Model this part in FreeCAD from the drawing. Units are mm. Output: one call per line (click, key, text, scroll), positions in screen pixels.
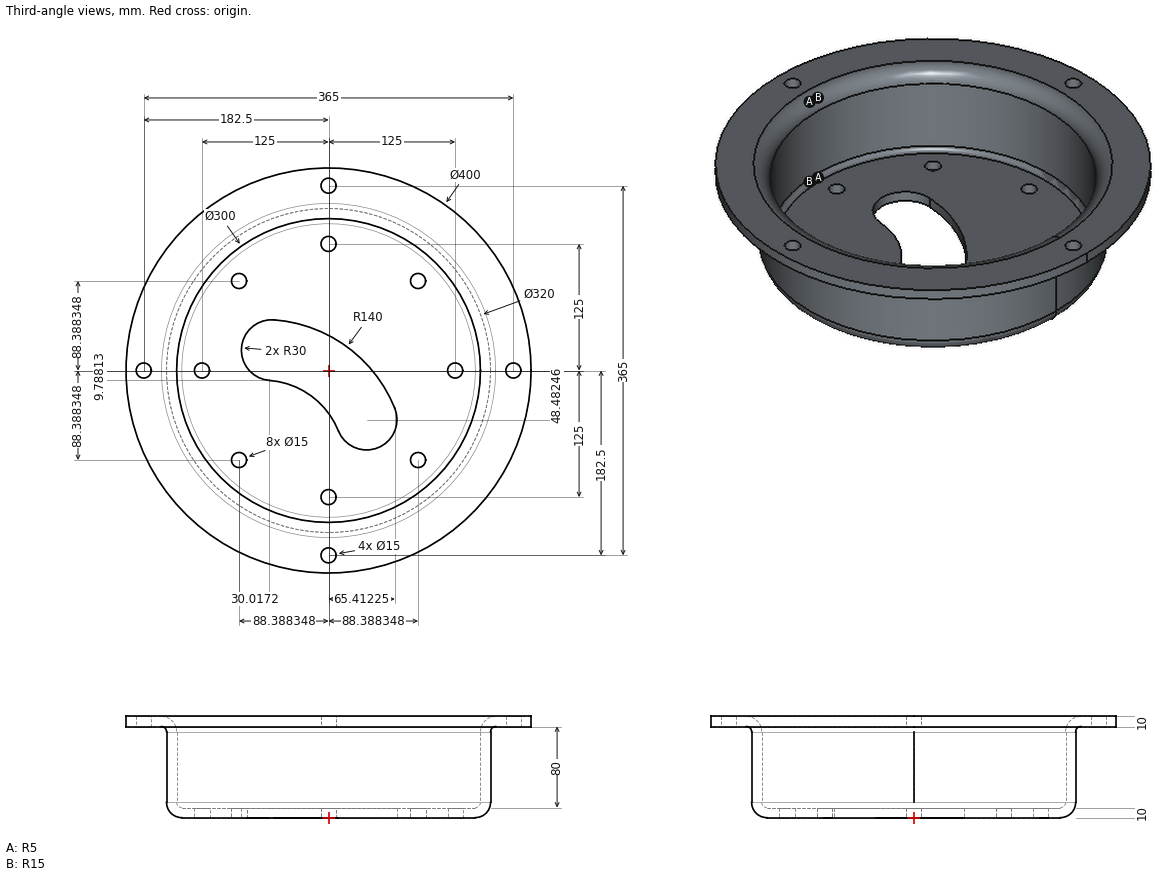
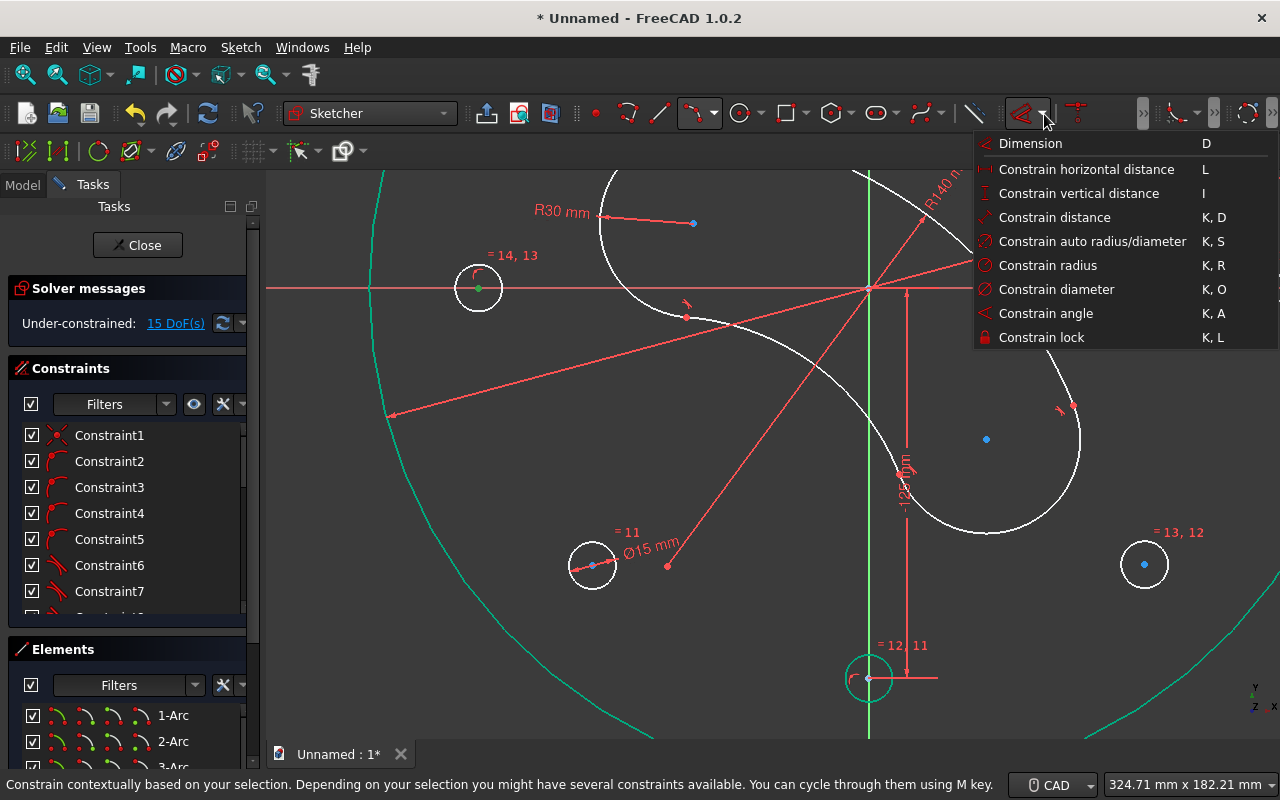
click(1126, 169)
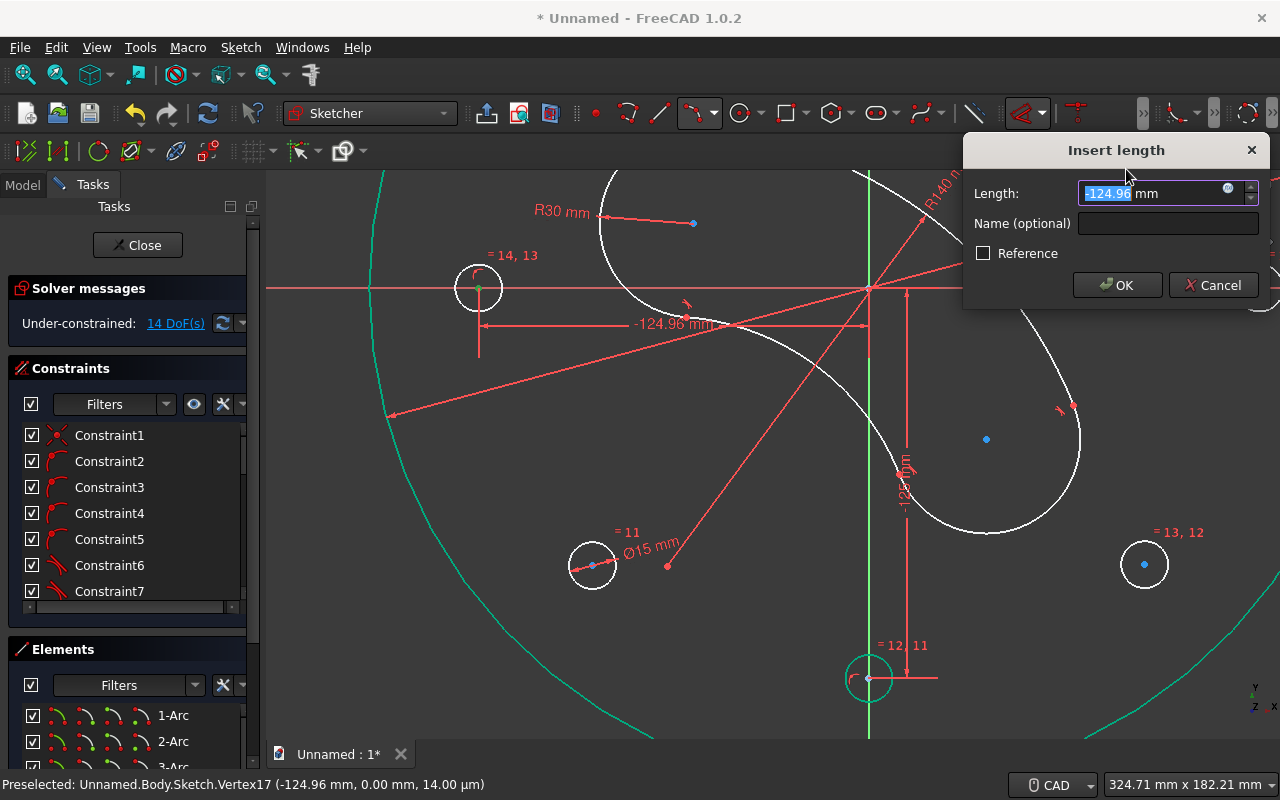
text(-125)
key(Return)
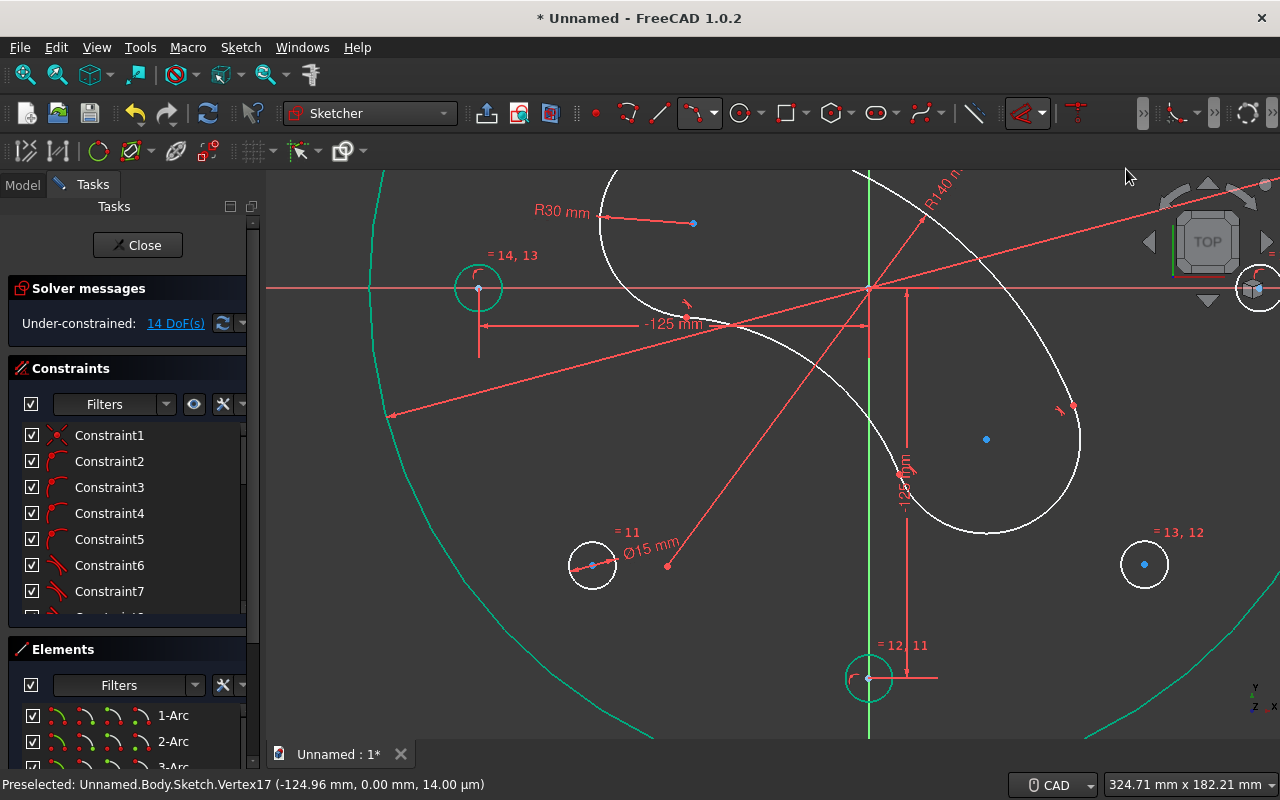
scroll(609, 551, down, 5)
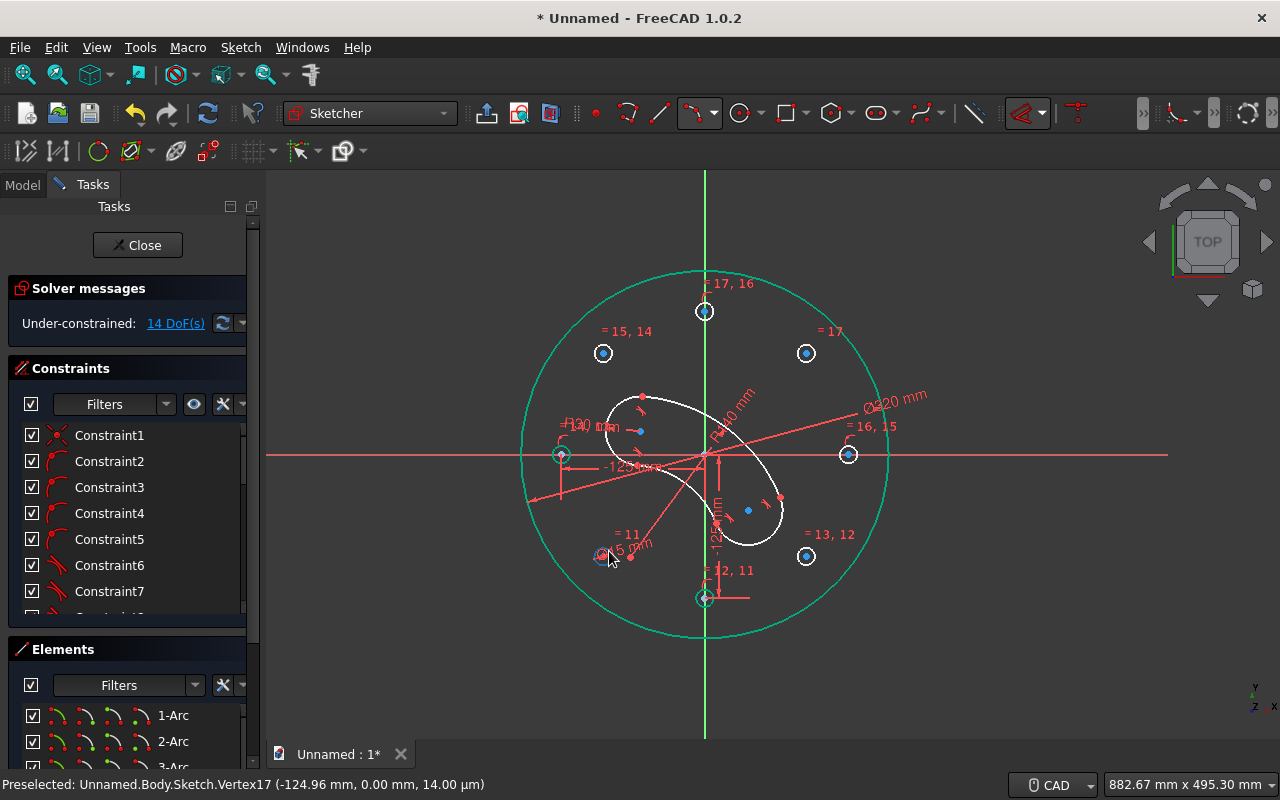
click(849, 455)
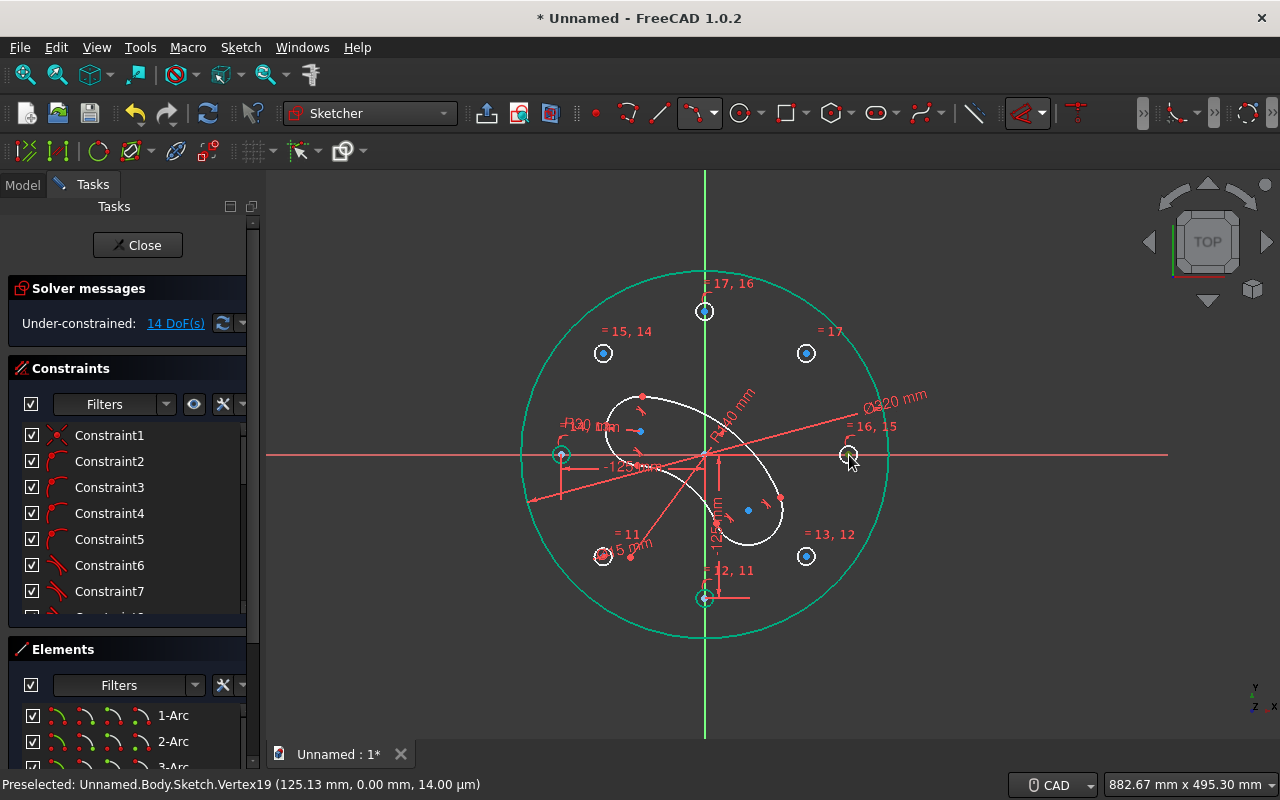
click(1044, 114)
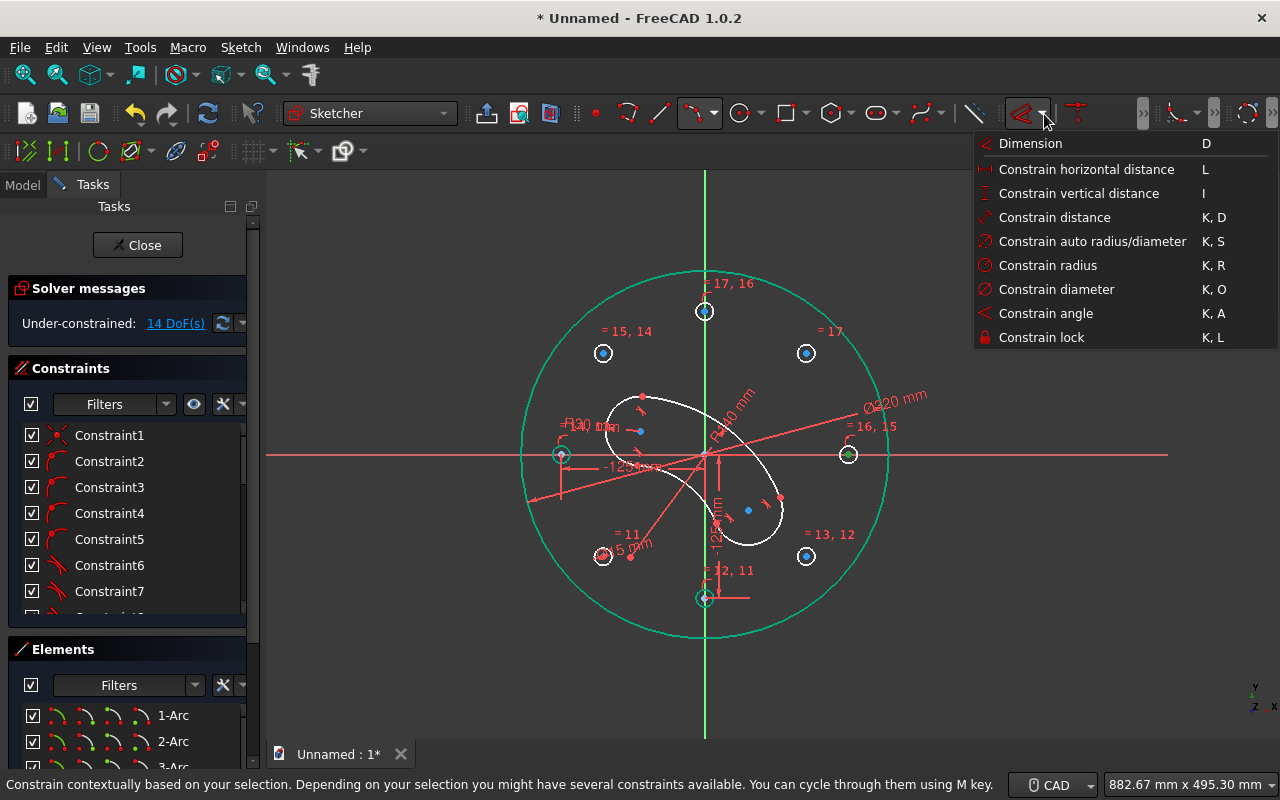
click(1126, 169)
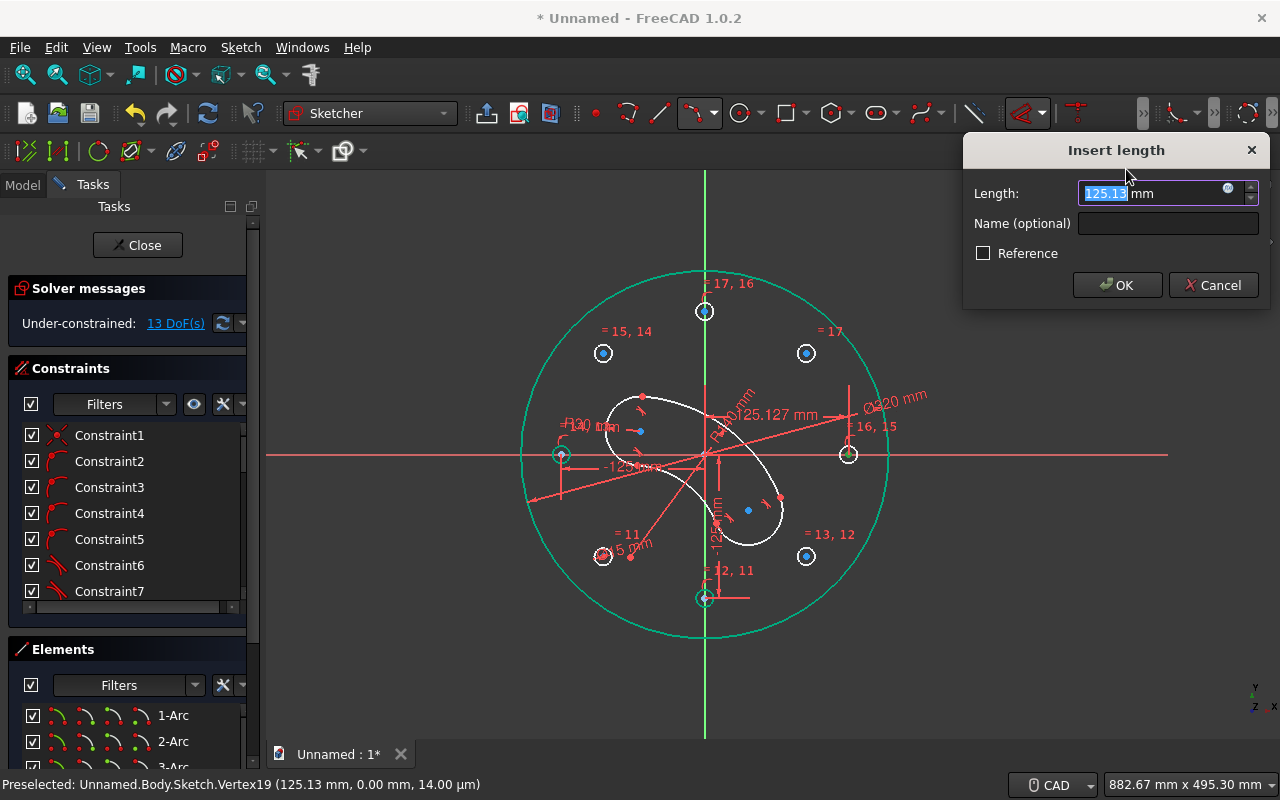
text(125)
key(Return)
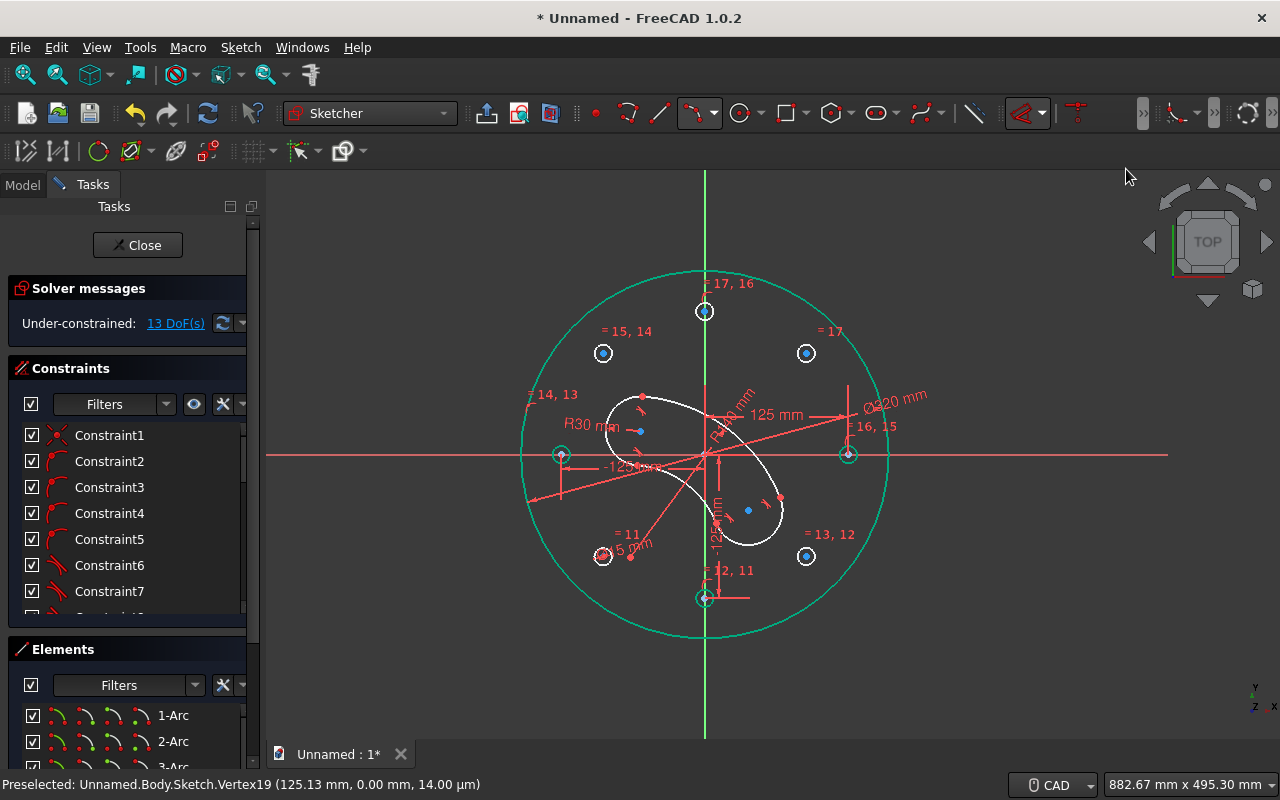
click(705, 312)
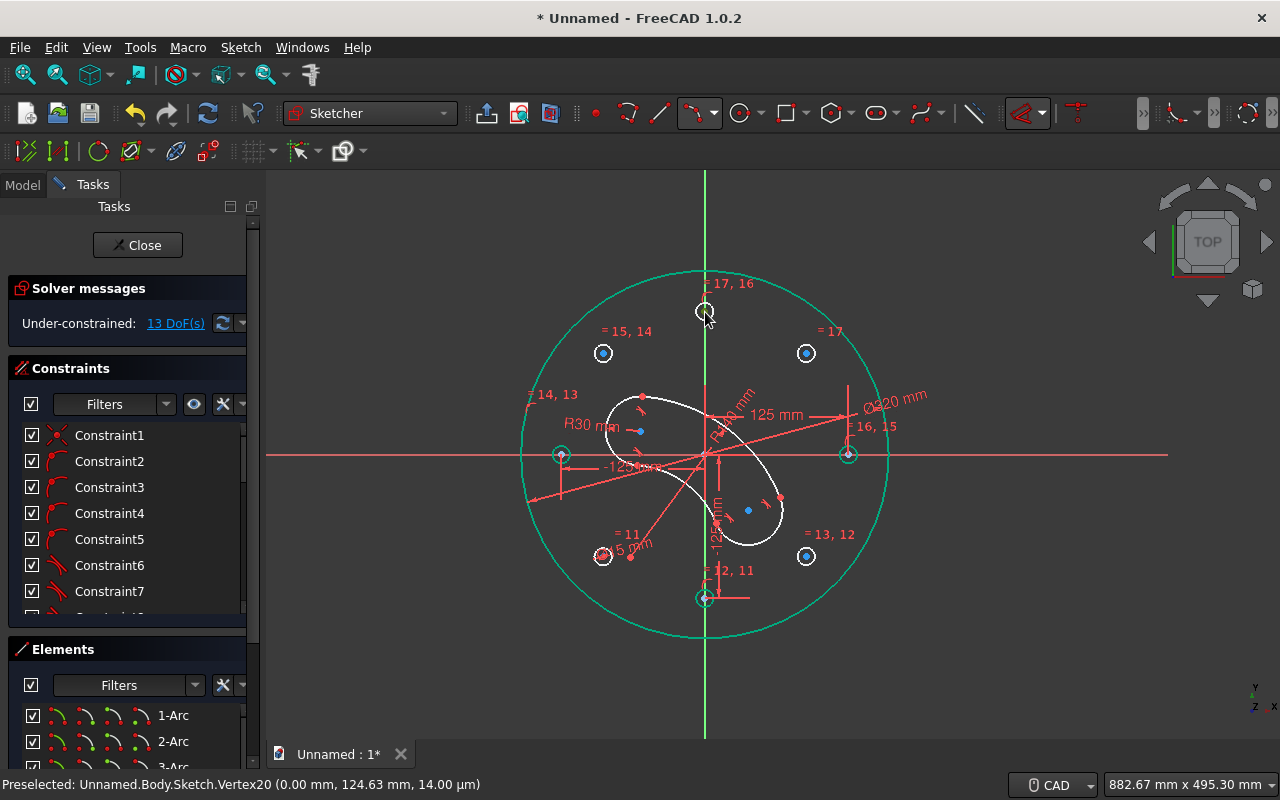
key(i)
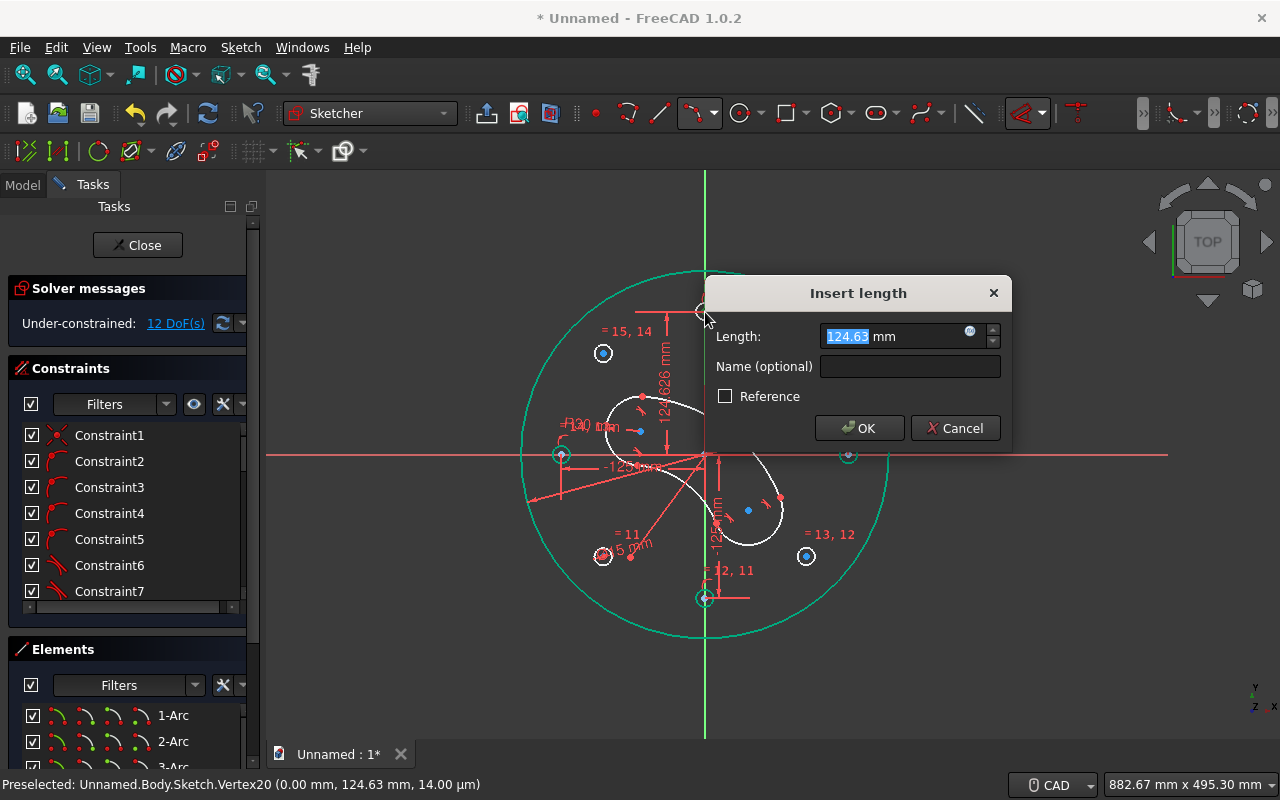
text(125)
key(Return)